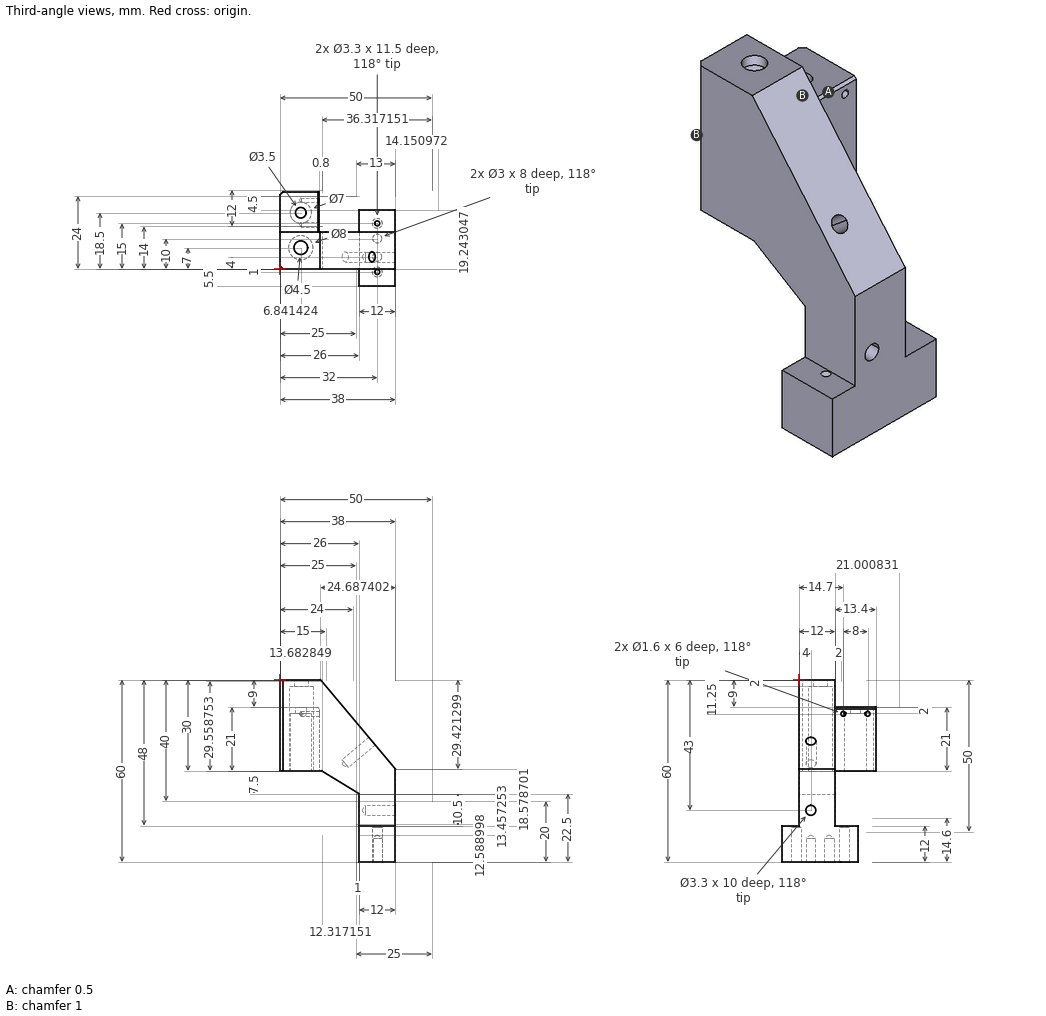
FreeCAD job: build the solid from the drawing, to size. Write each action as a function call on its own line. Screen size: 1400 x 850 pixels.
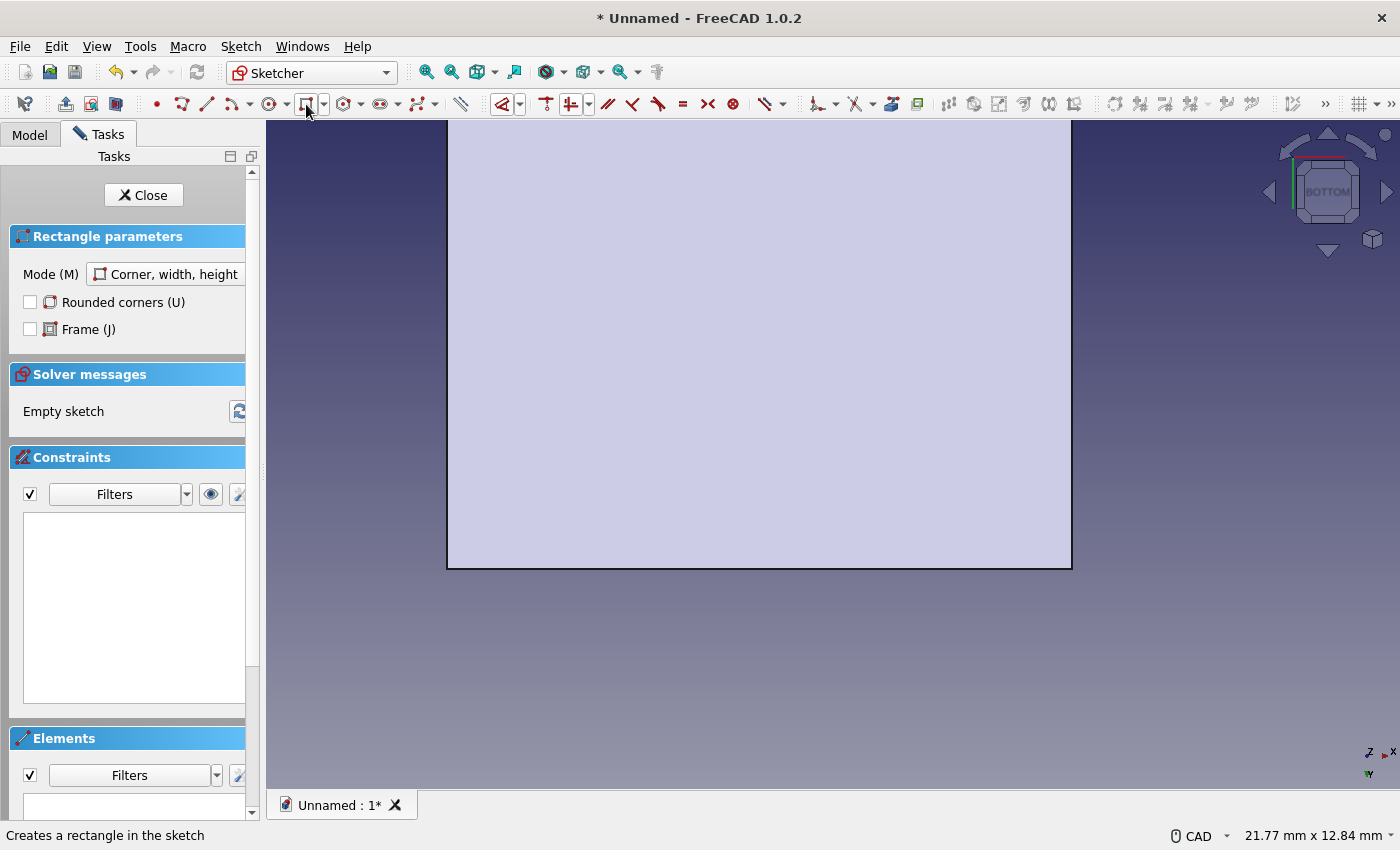
click(447, 335)
click(1072, 569)
key(Escape)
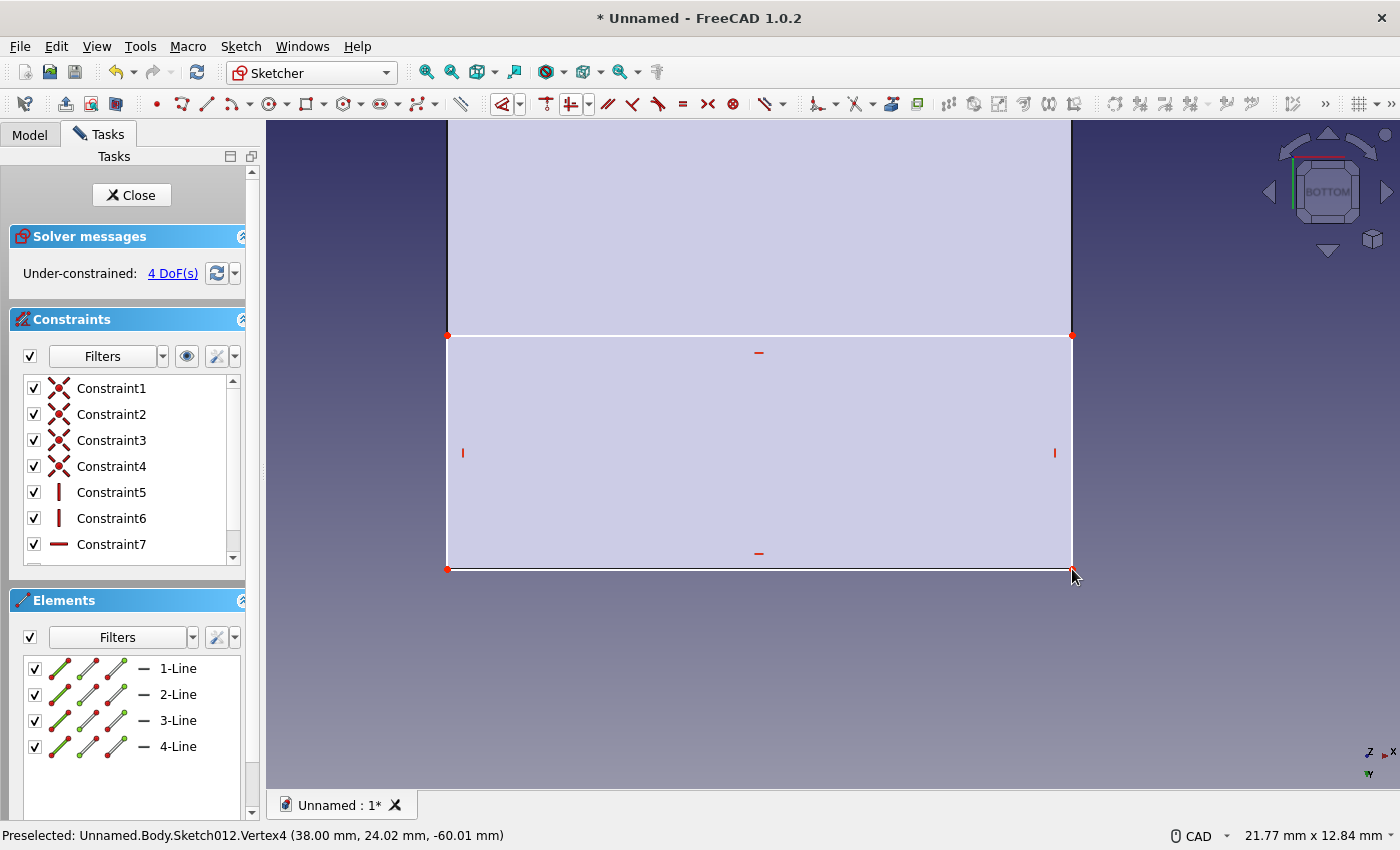
click(635, 570)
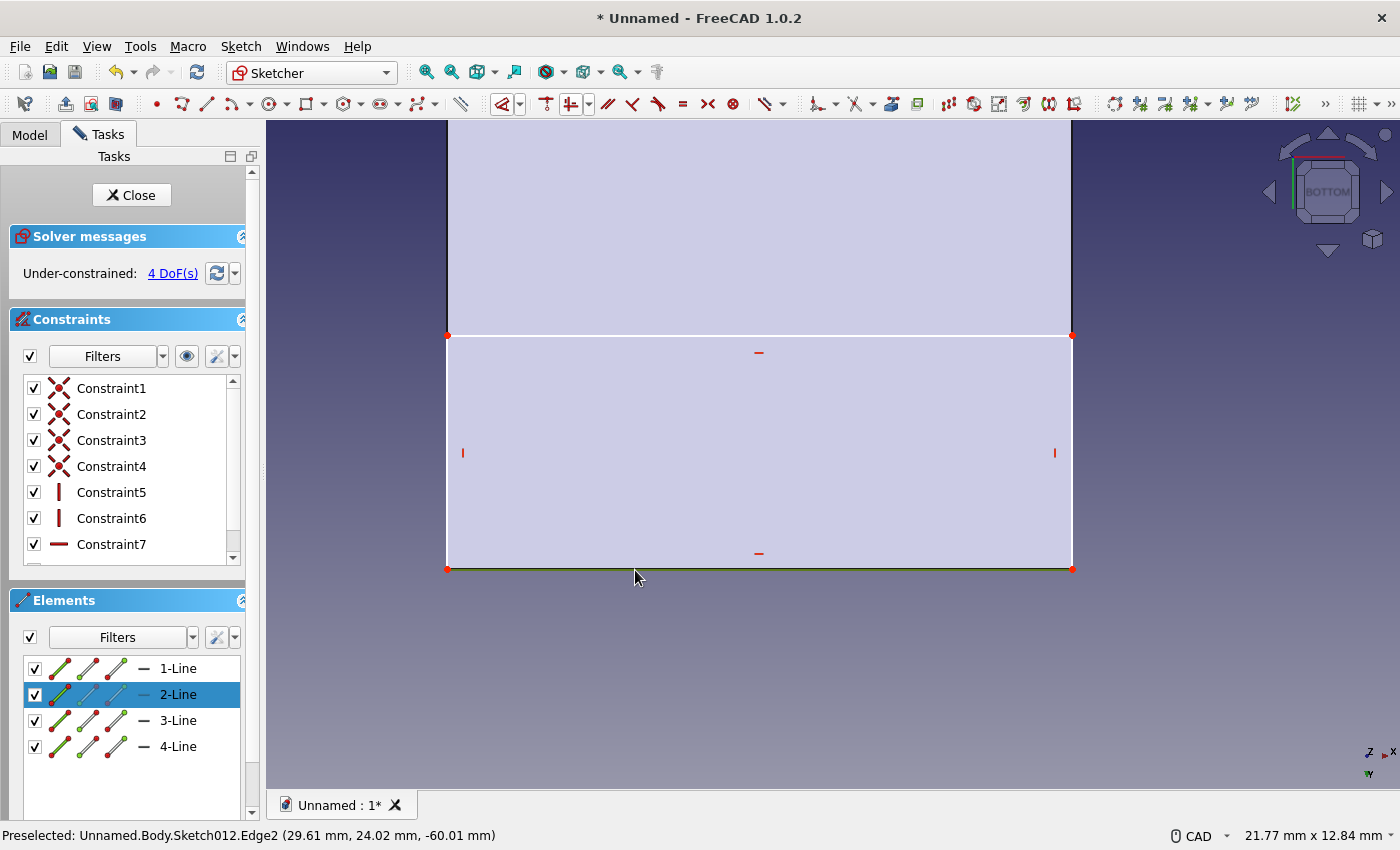
click(520, 104)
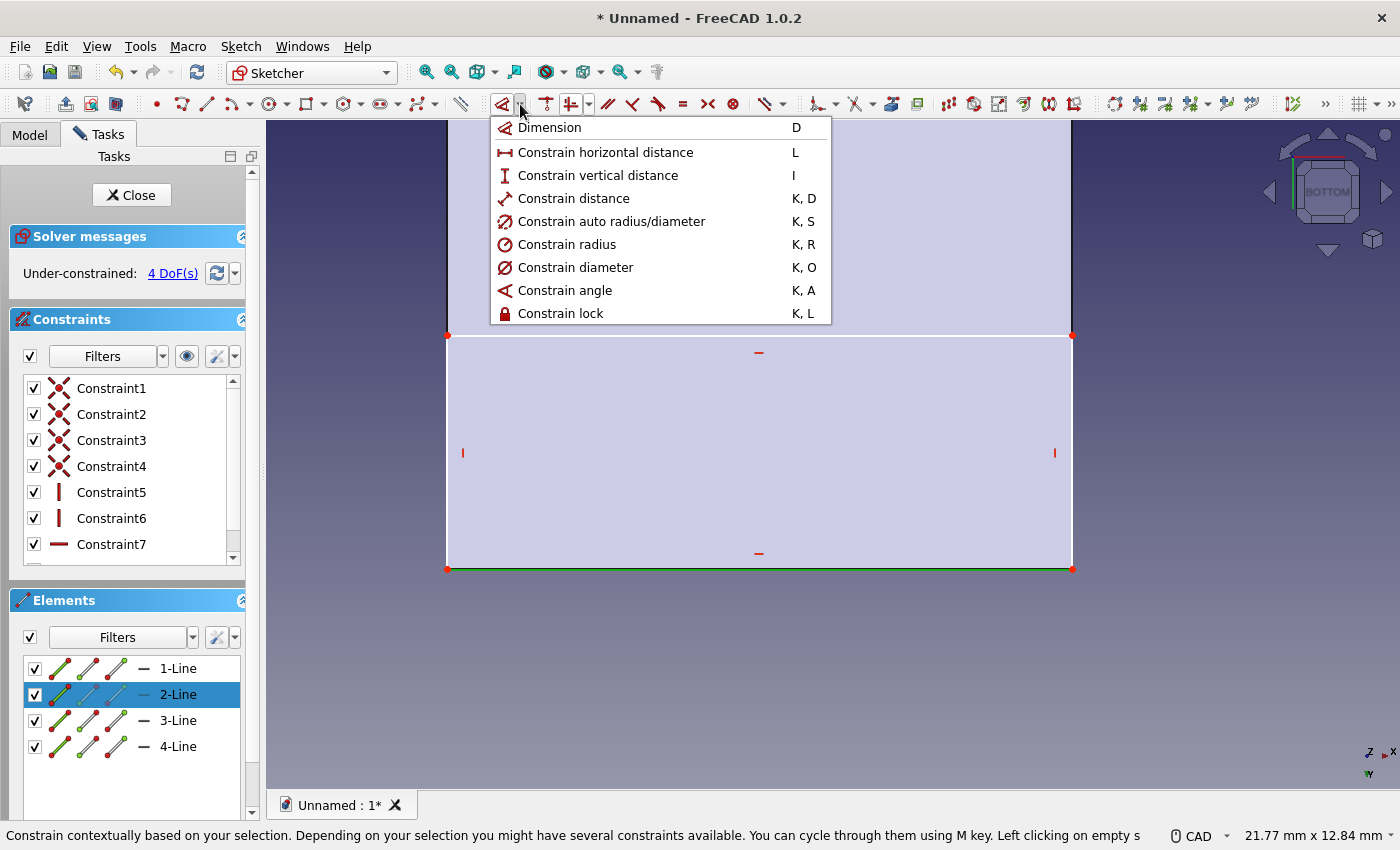
click(661, 152)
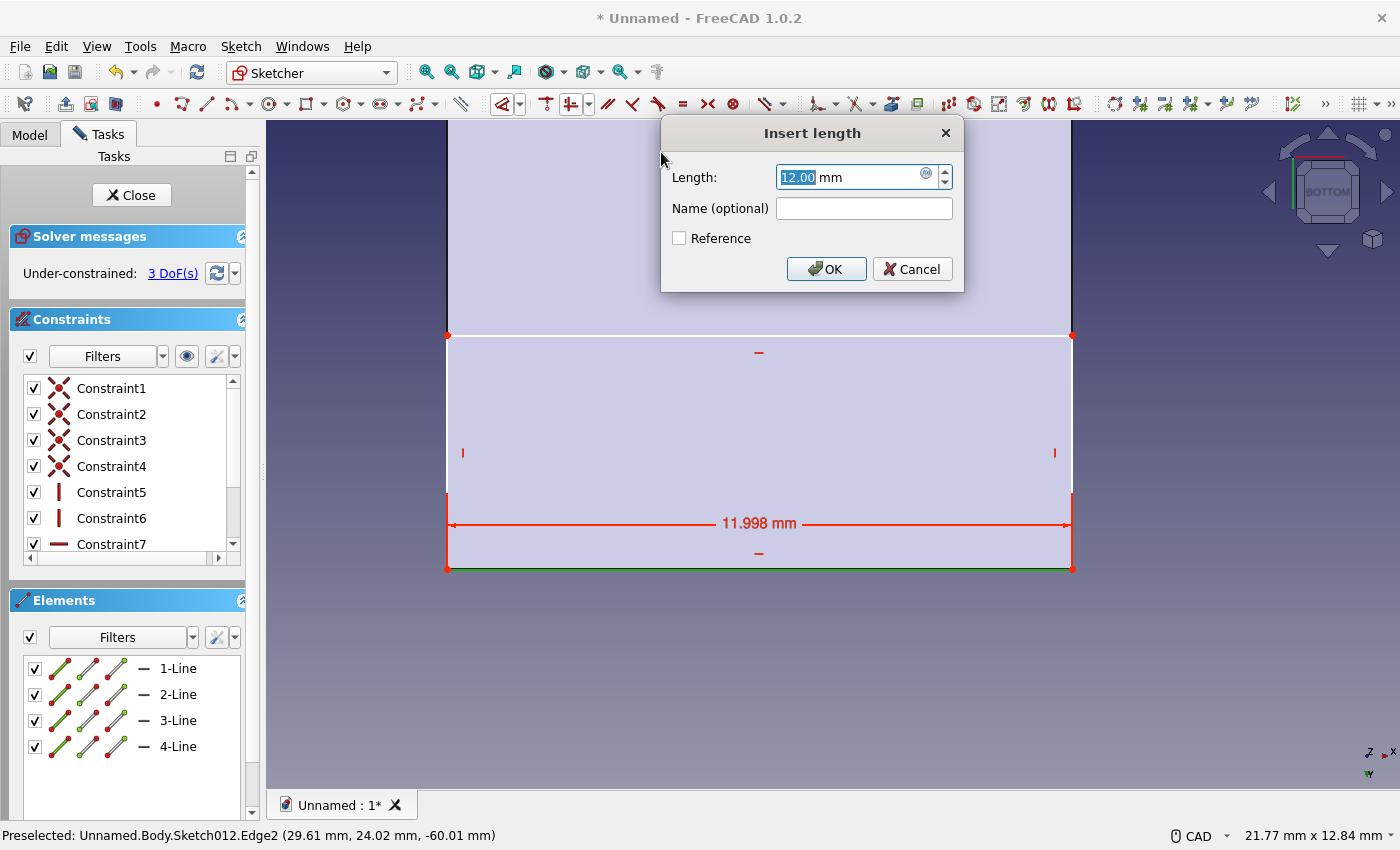
text(12)
key(Return)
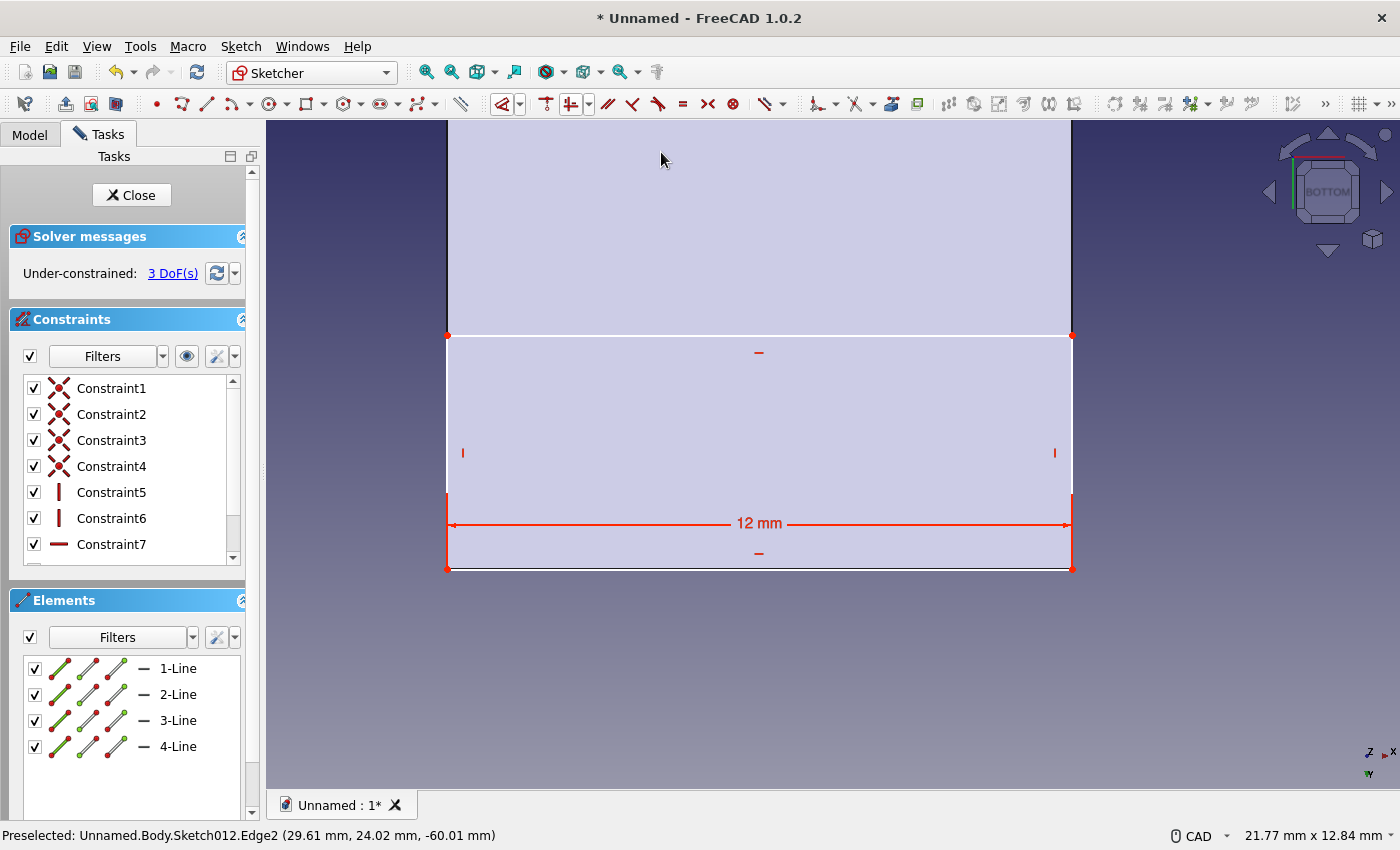
click(447, 406)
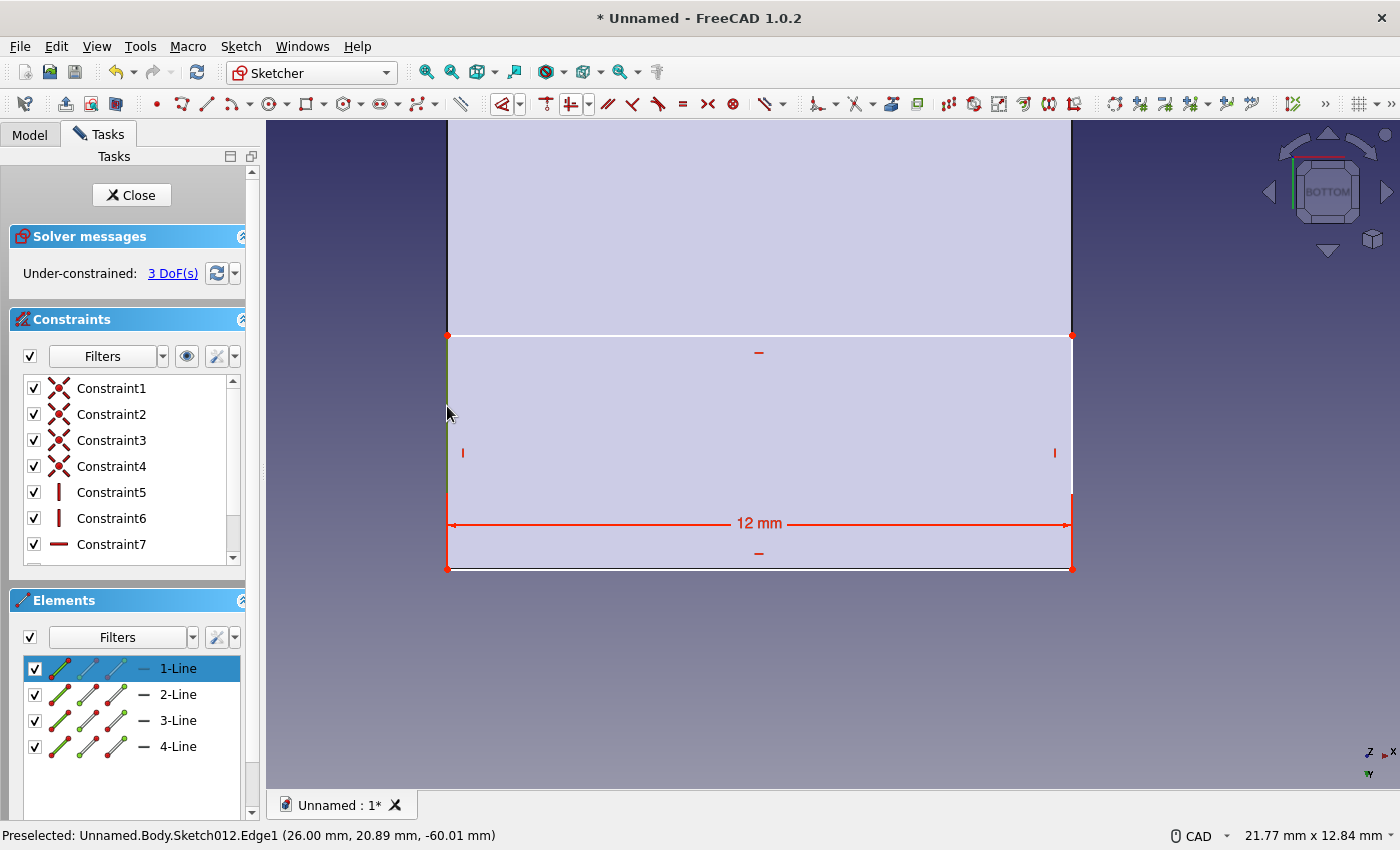
key(i)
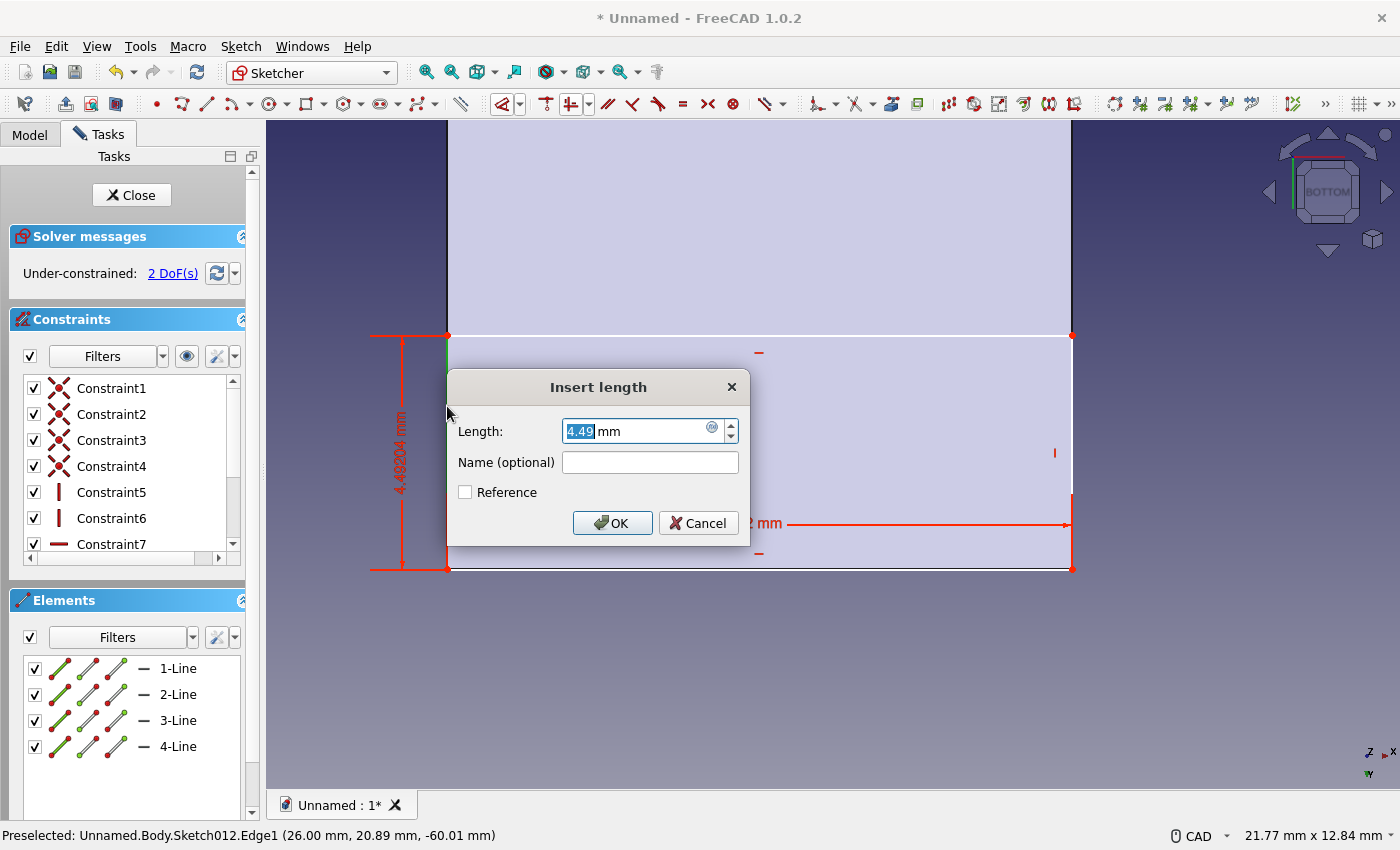
text(4.5)
key(Return)